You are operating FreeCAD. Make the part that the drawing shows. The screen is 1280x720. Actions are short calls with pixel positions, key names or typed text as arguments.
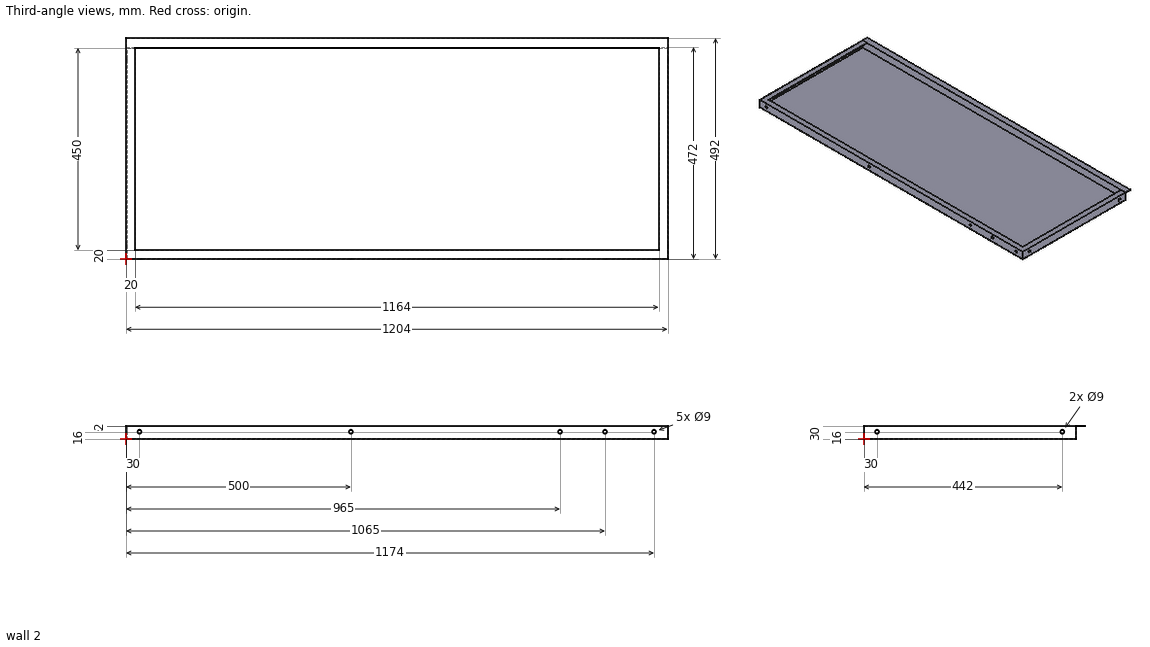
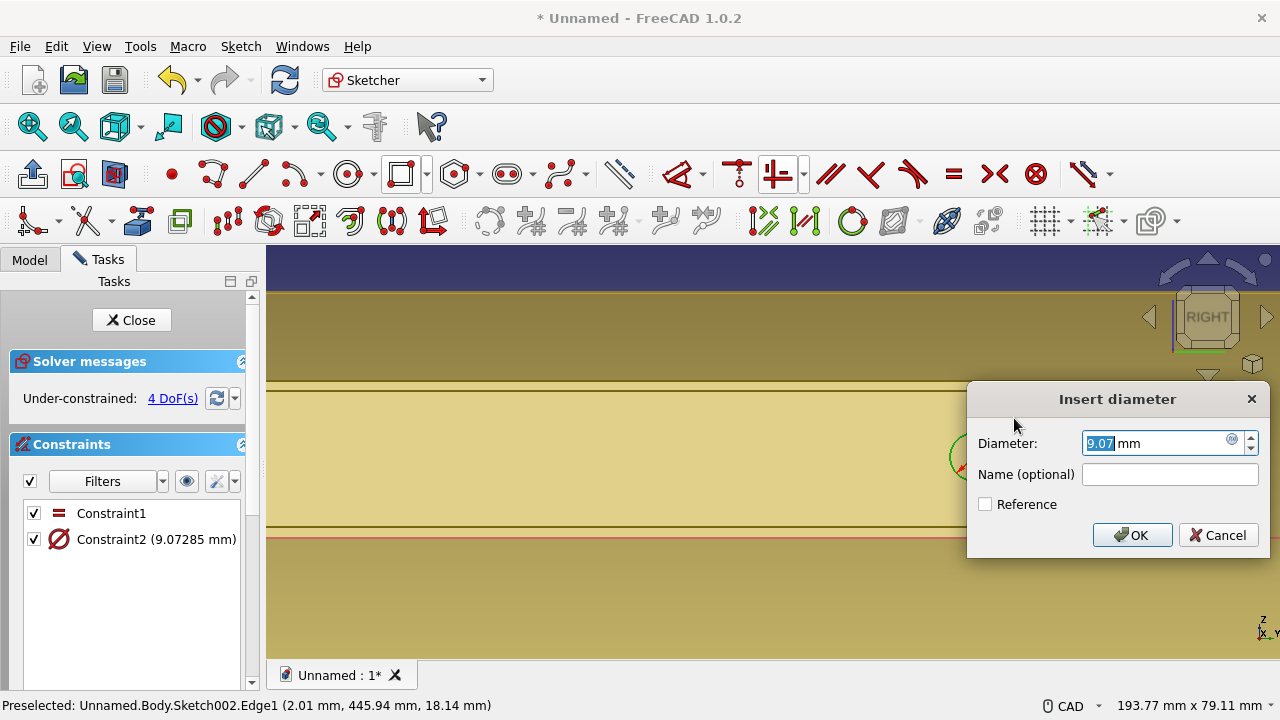
text(9)
key(Return)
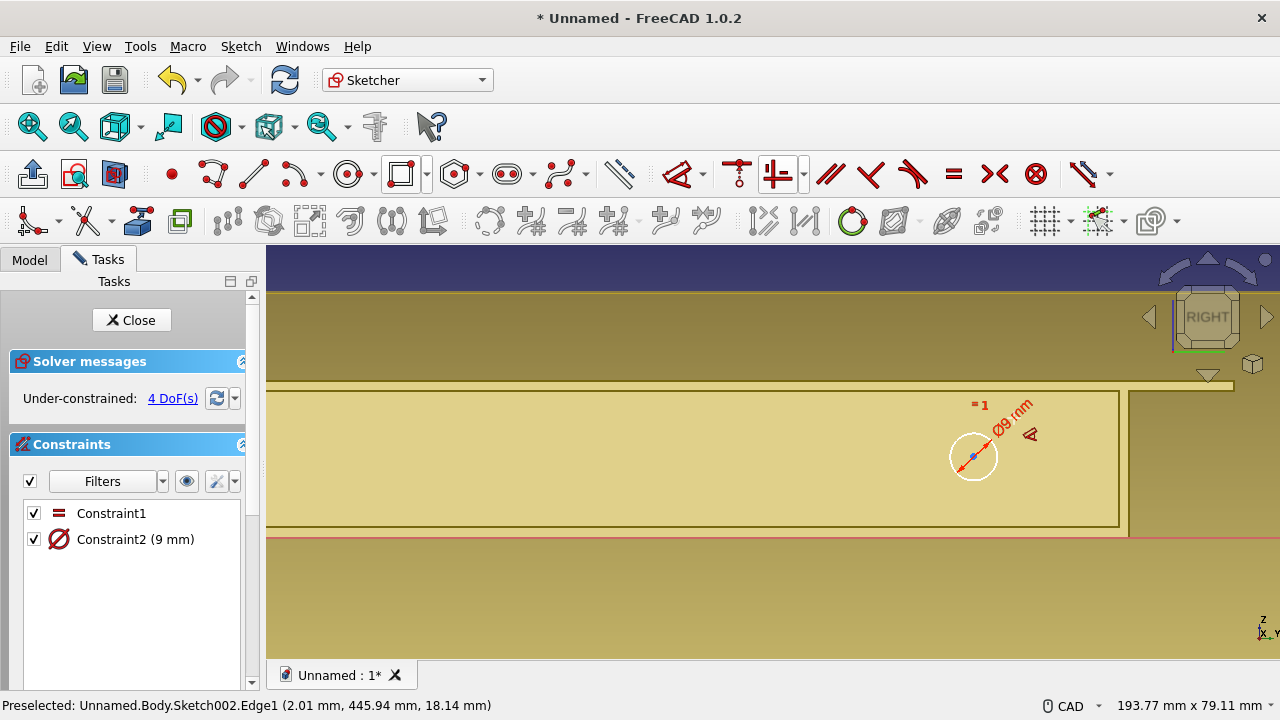
click(974, 457)
click(1008, 497)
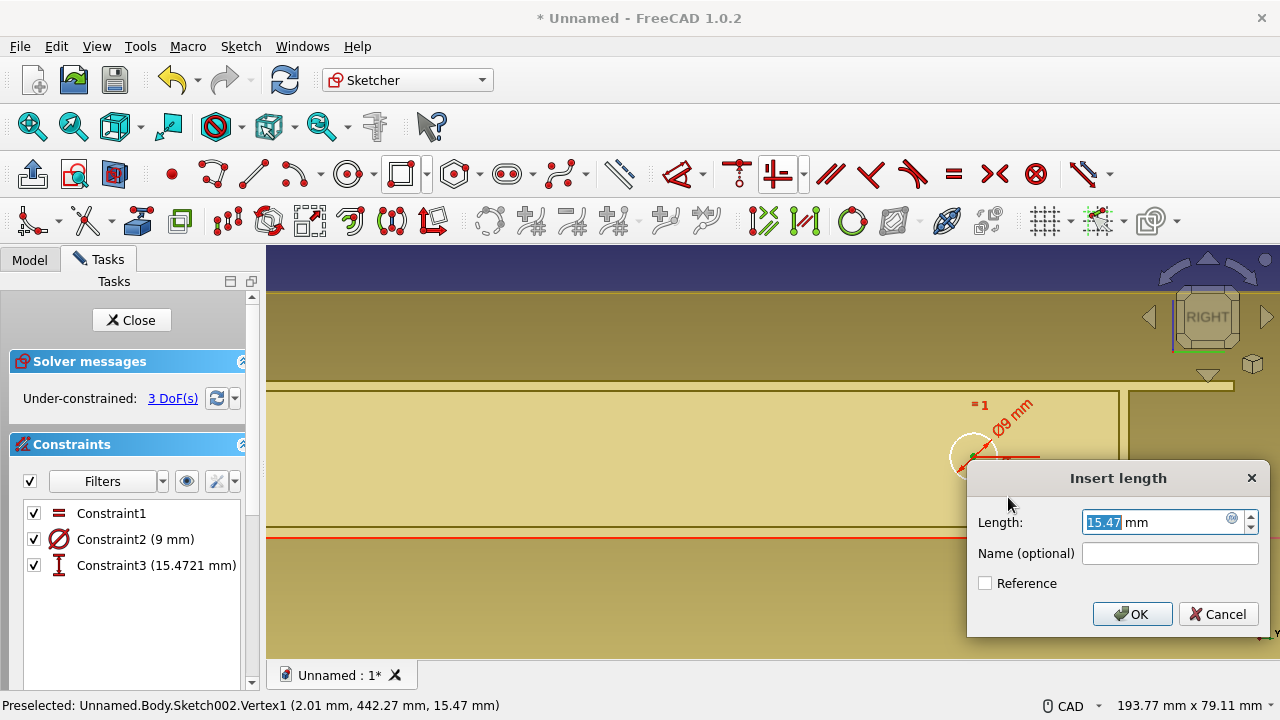
text(16)
key(Return)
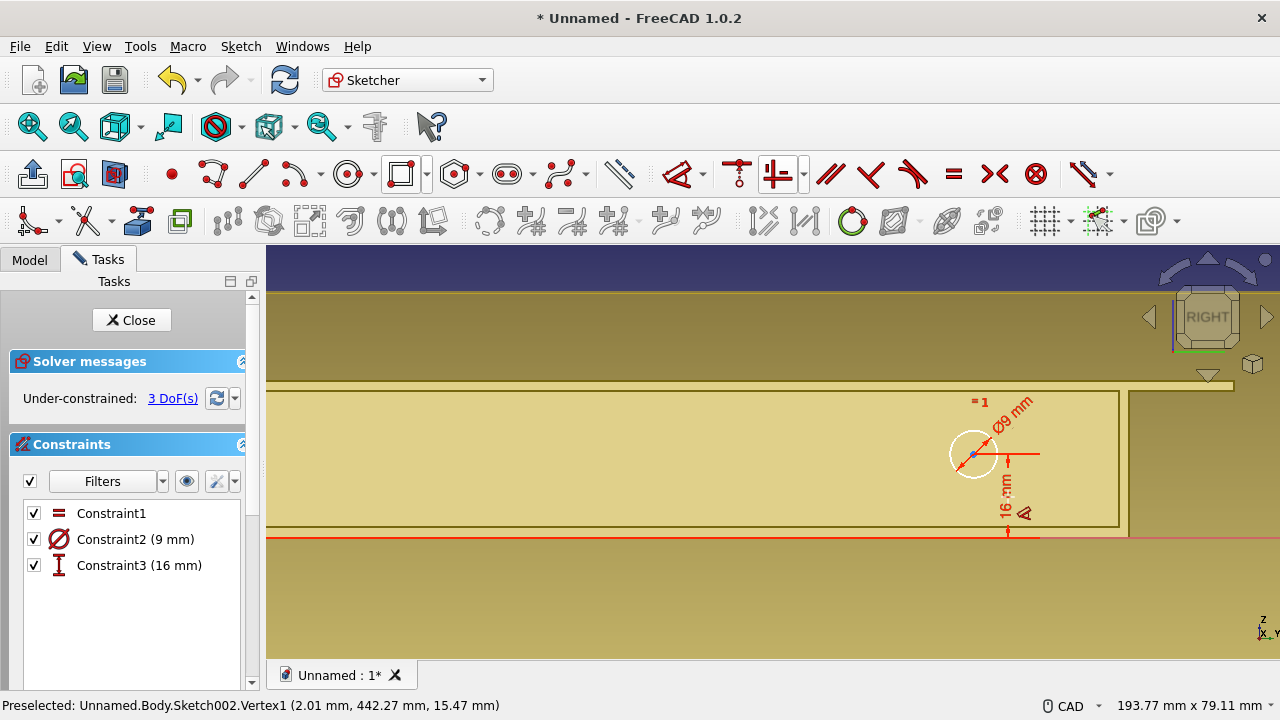
scroll(991, 441, down, 7)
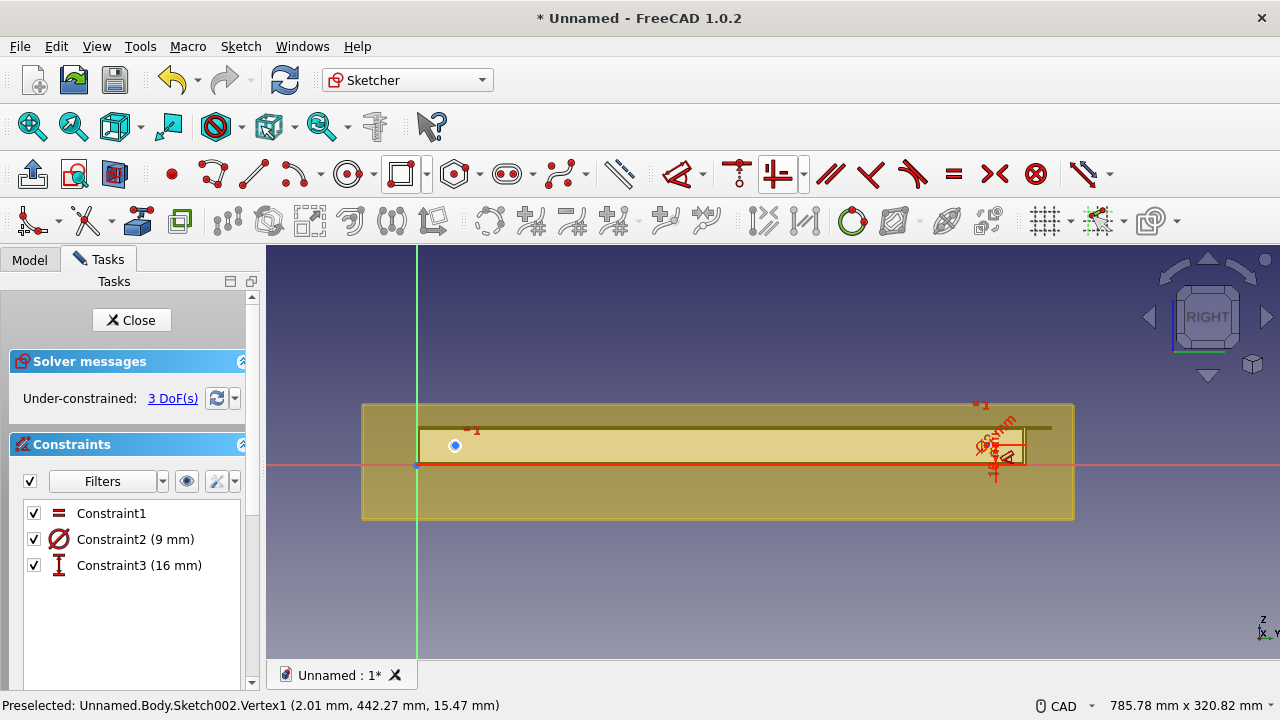
click(455, 446)
click(436, 499)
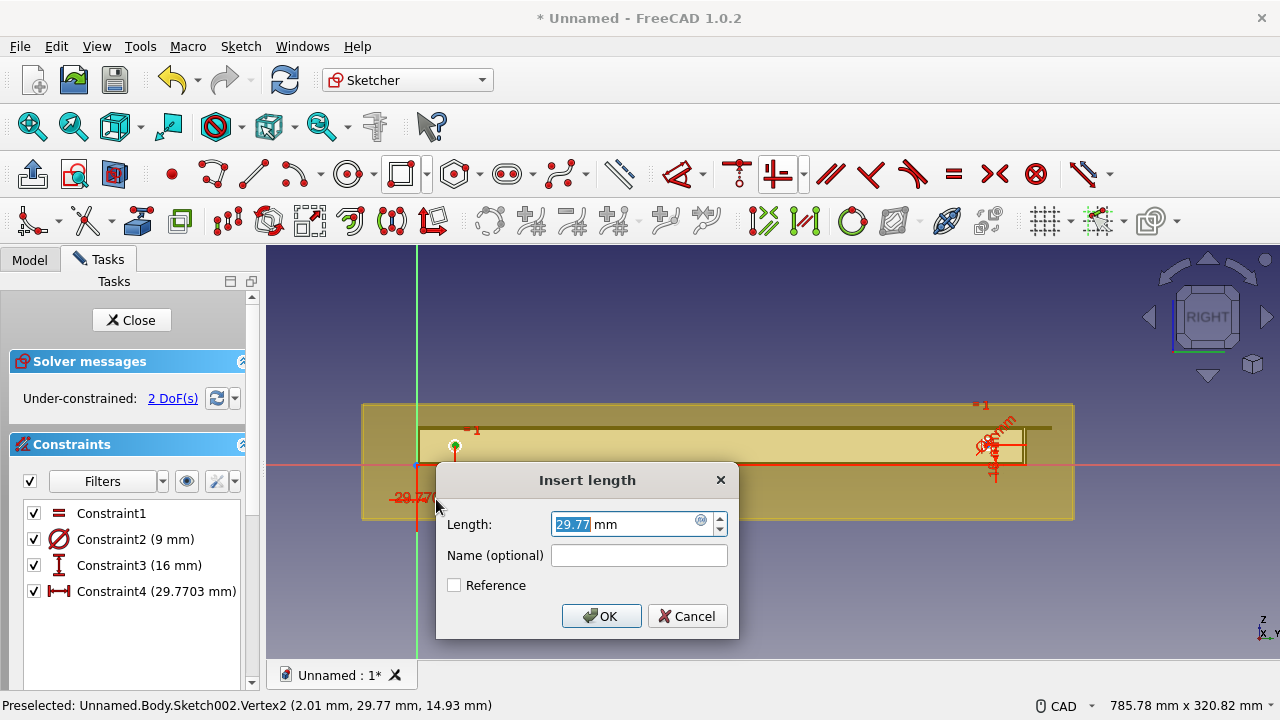
text(30)
key(Return)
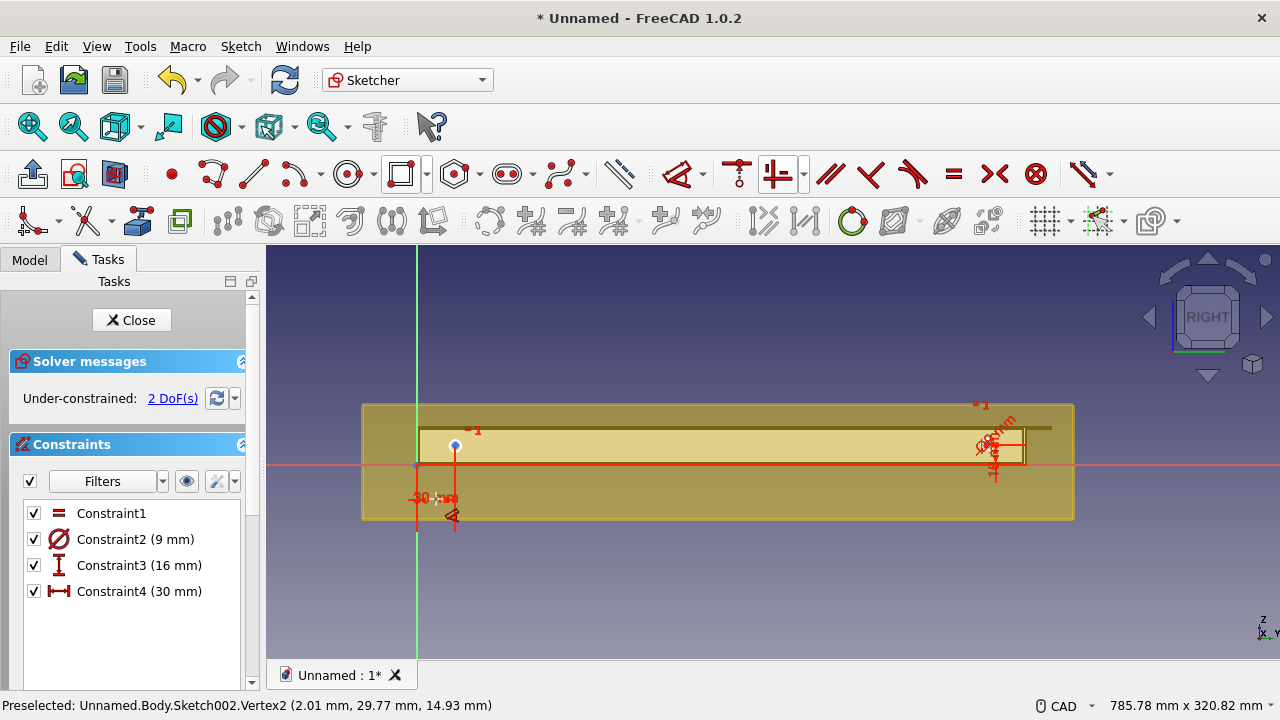
scroll(455, 446, up, 4)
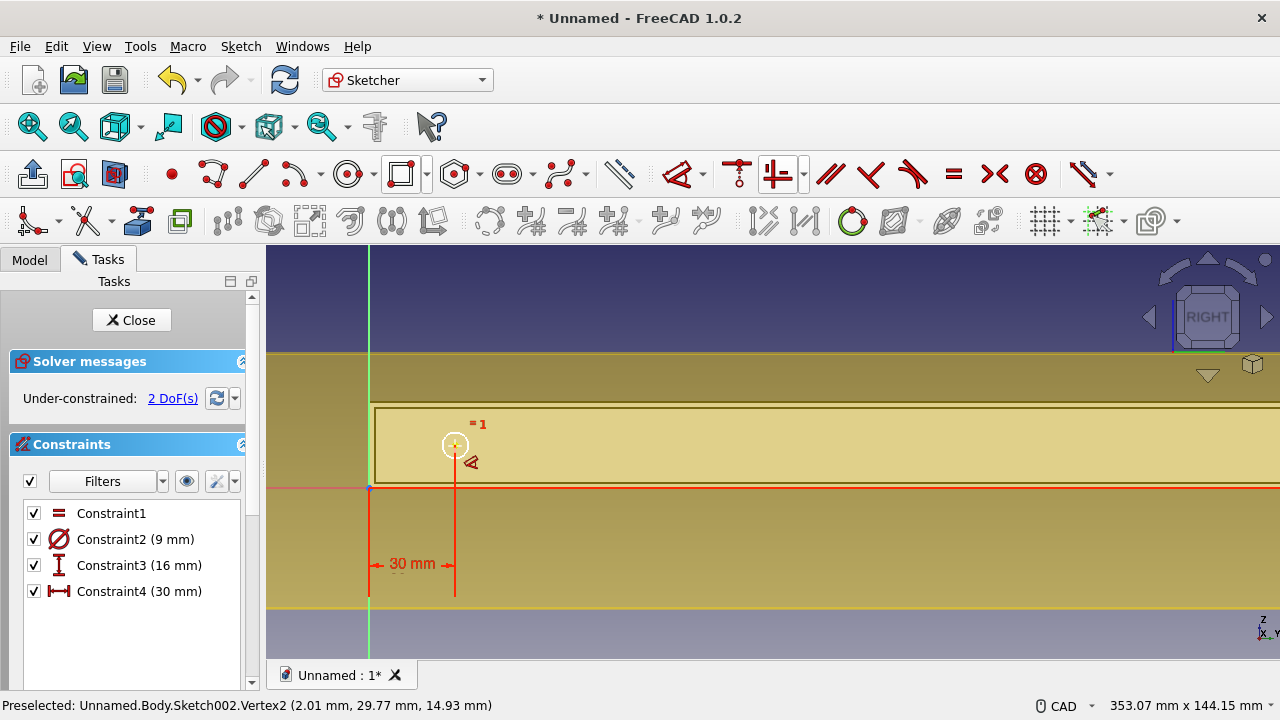
click(455, 445)
click(335, 467)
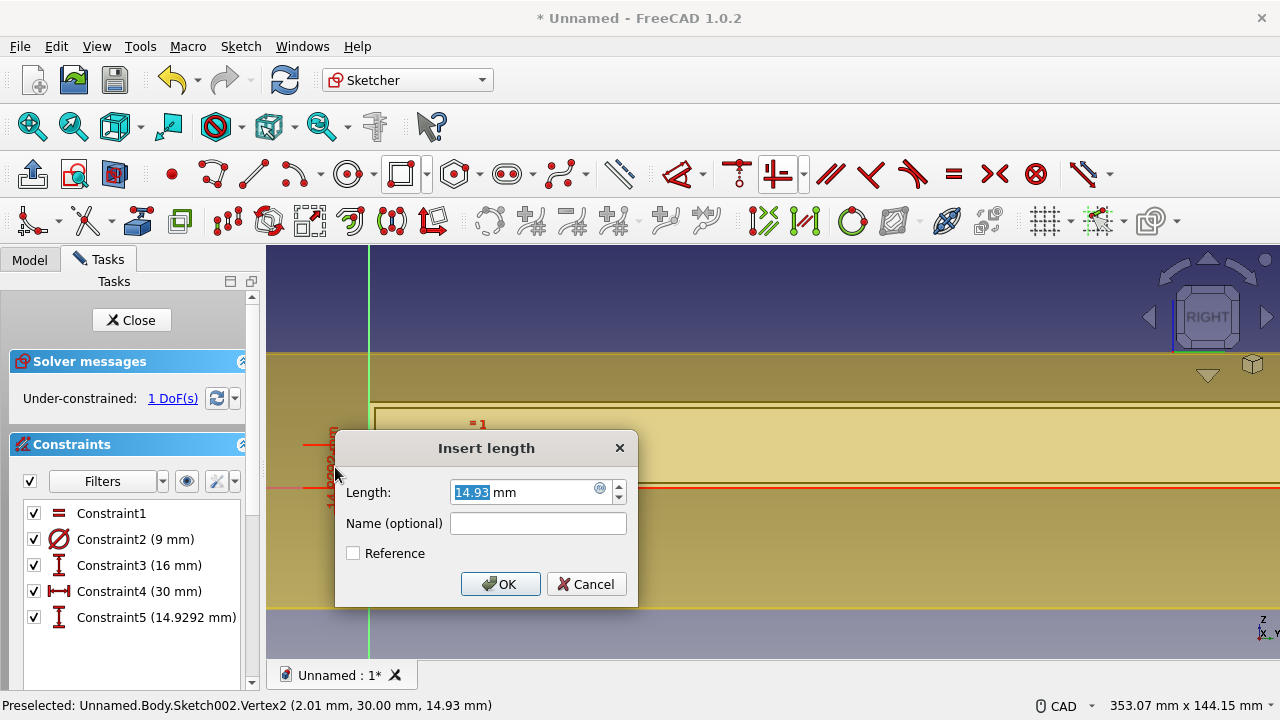
text(16)
key(Return)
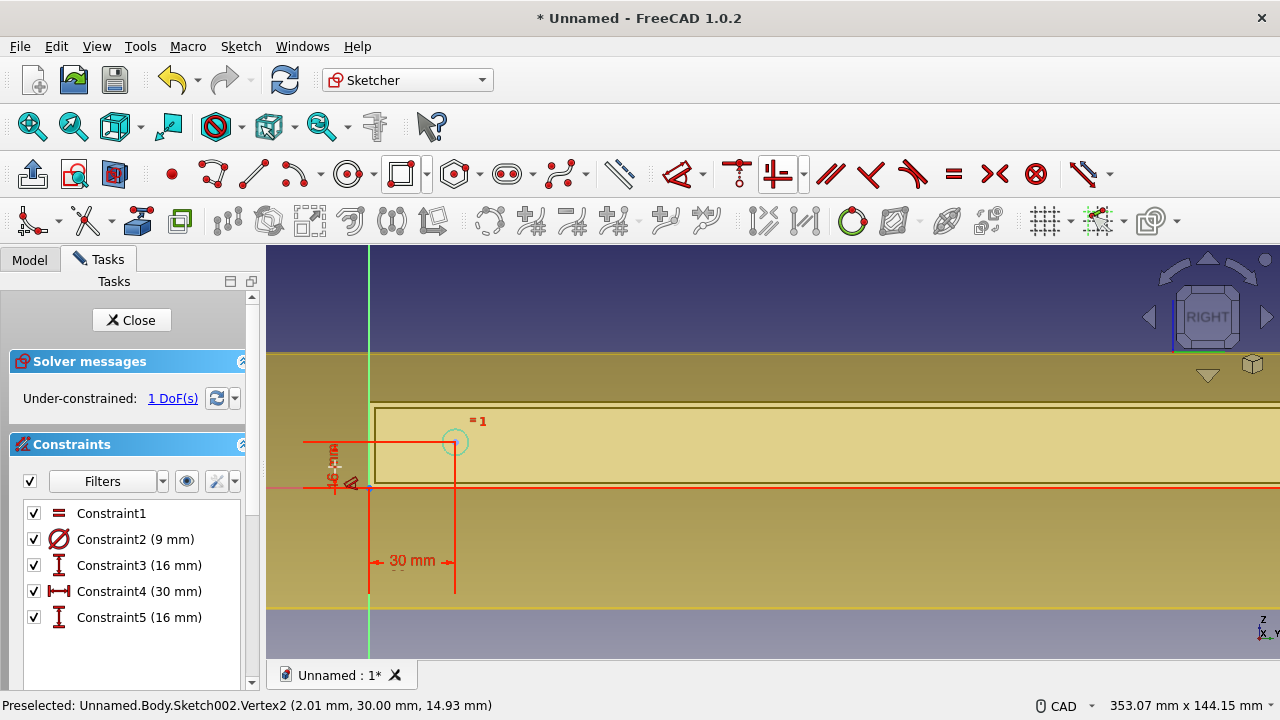
scroll(455, 446, down, 4)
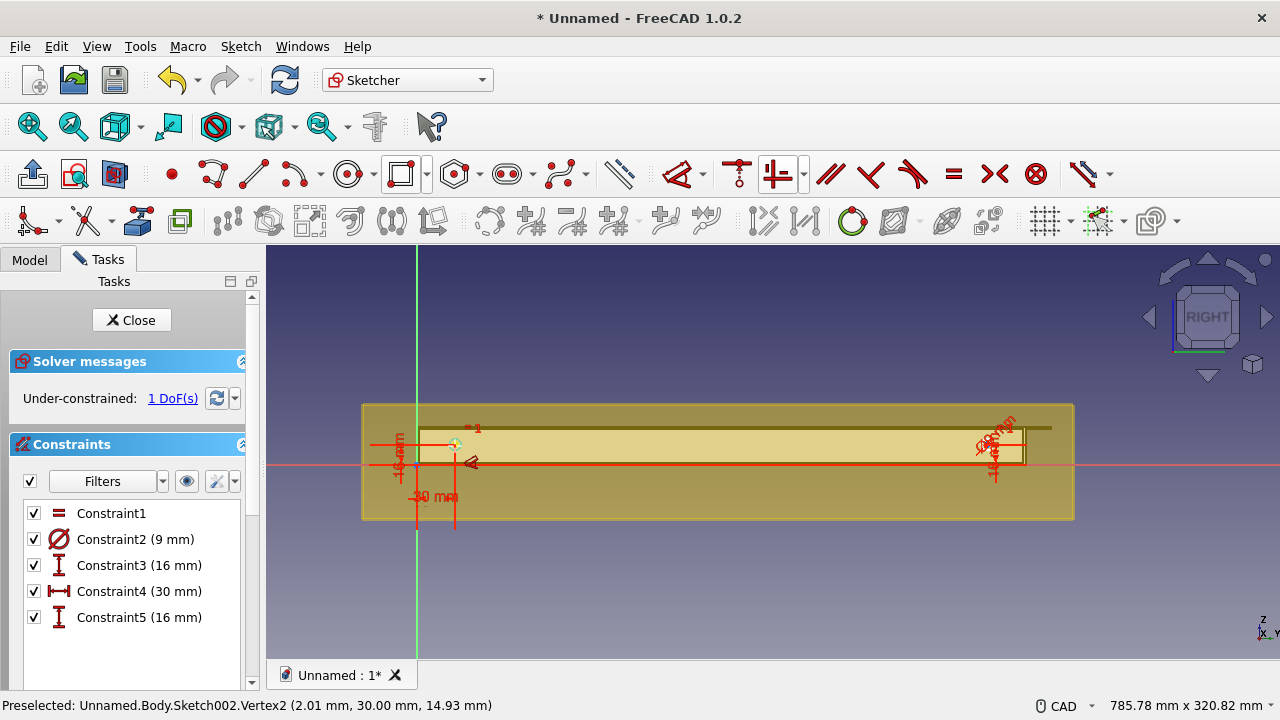
click(987, 445)
click(702, 499)